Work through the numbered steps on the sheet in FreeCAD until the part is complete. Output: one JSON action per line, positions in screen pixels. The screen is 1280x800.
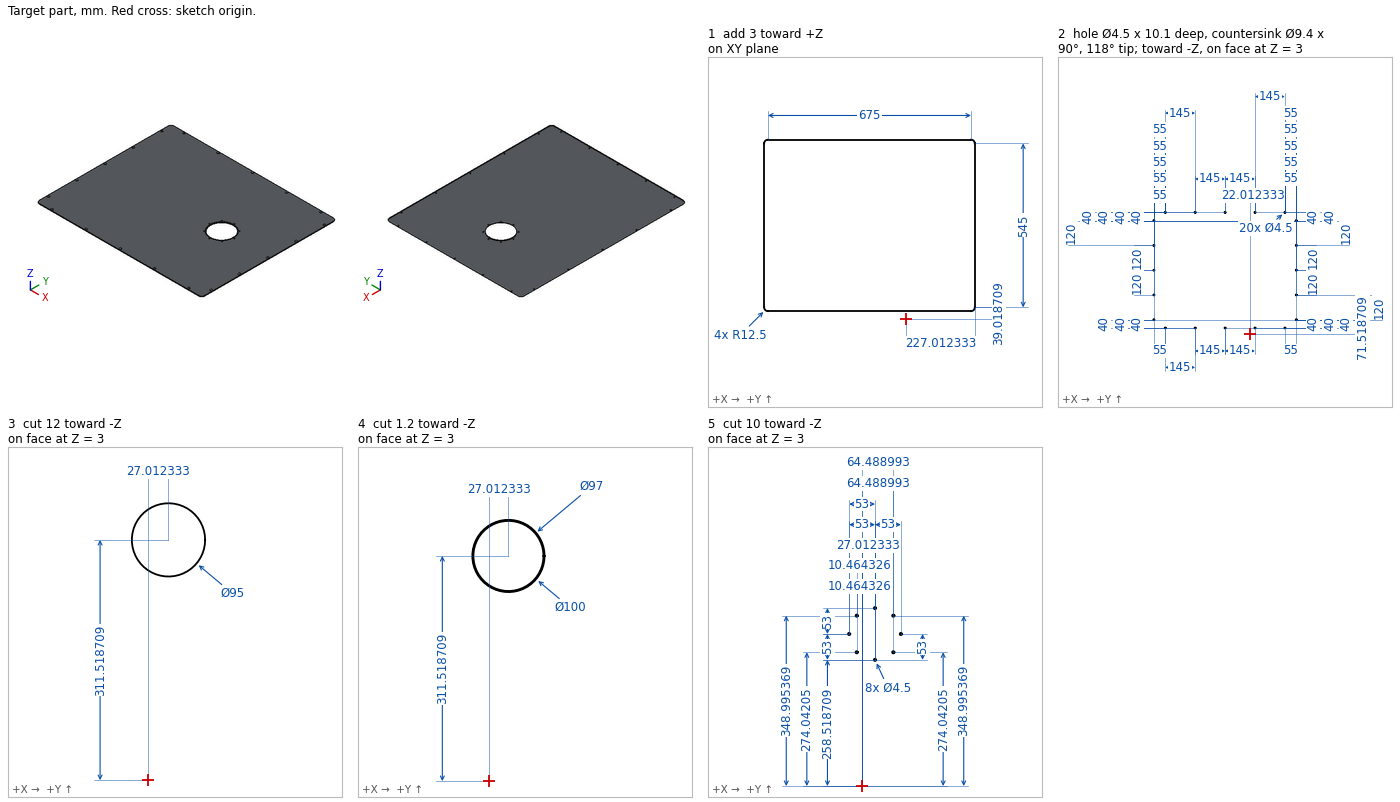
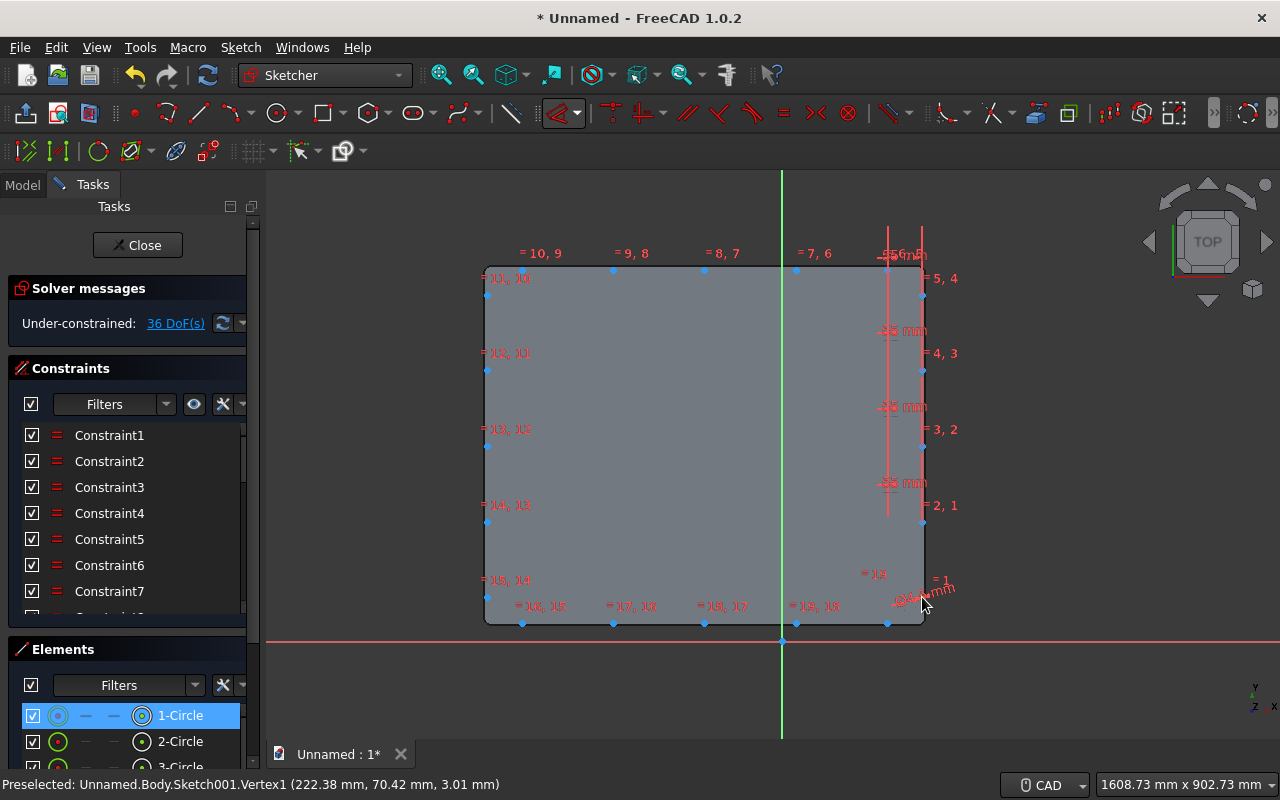
{"action": "left_click", "coordinate": [888, 270]}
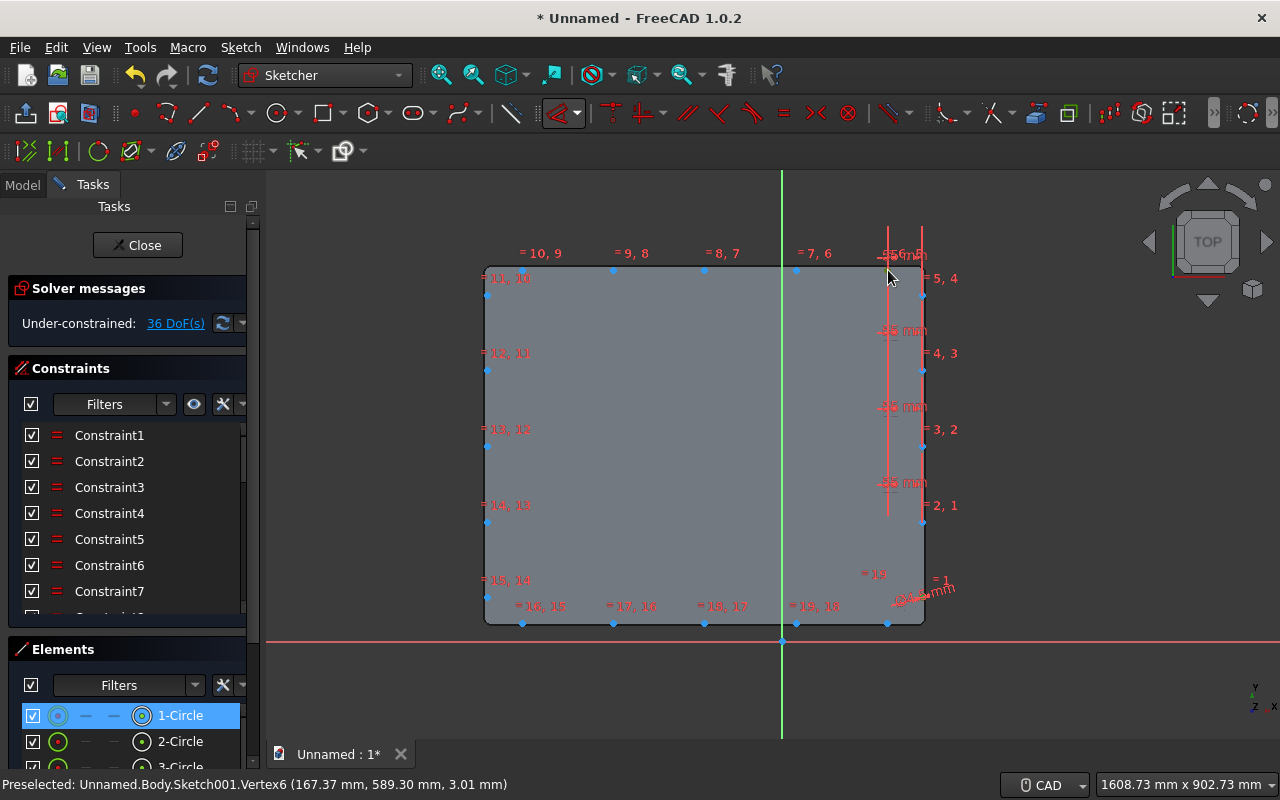
{"action": "key", "text": "l"}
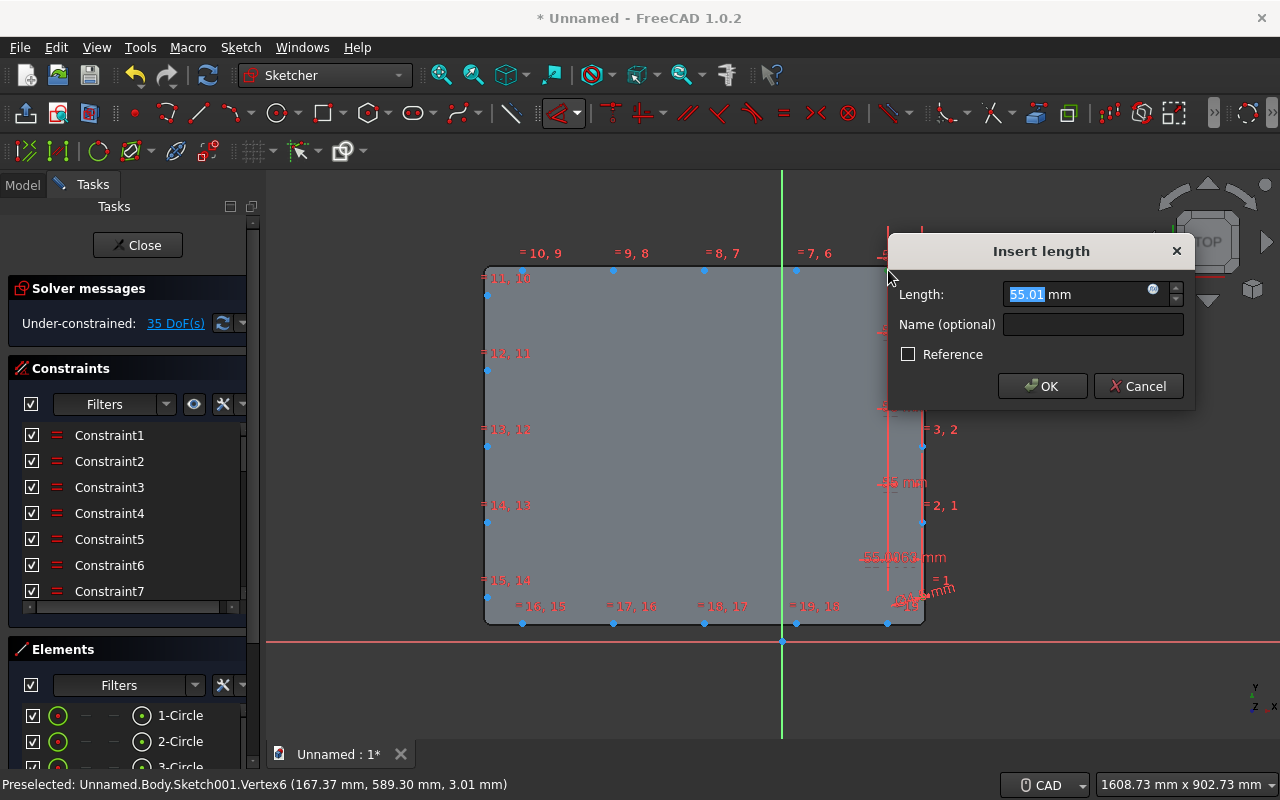
{"action": "type", "text": "55"}
{"action": "key", "text": "Return"}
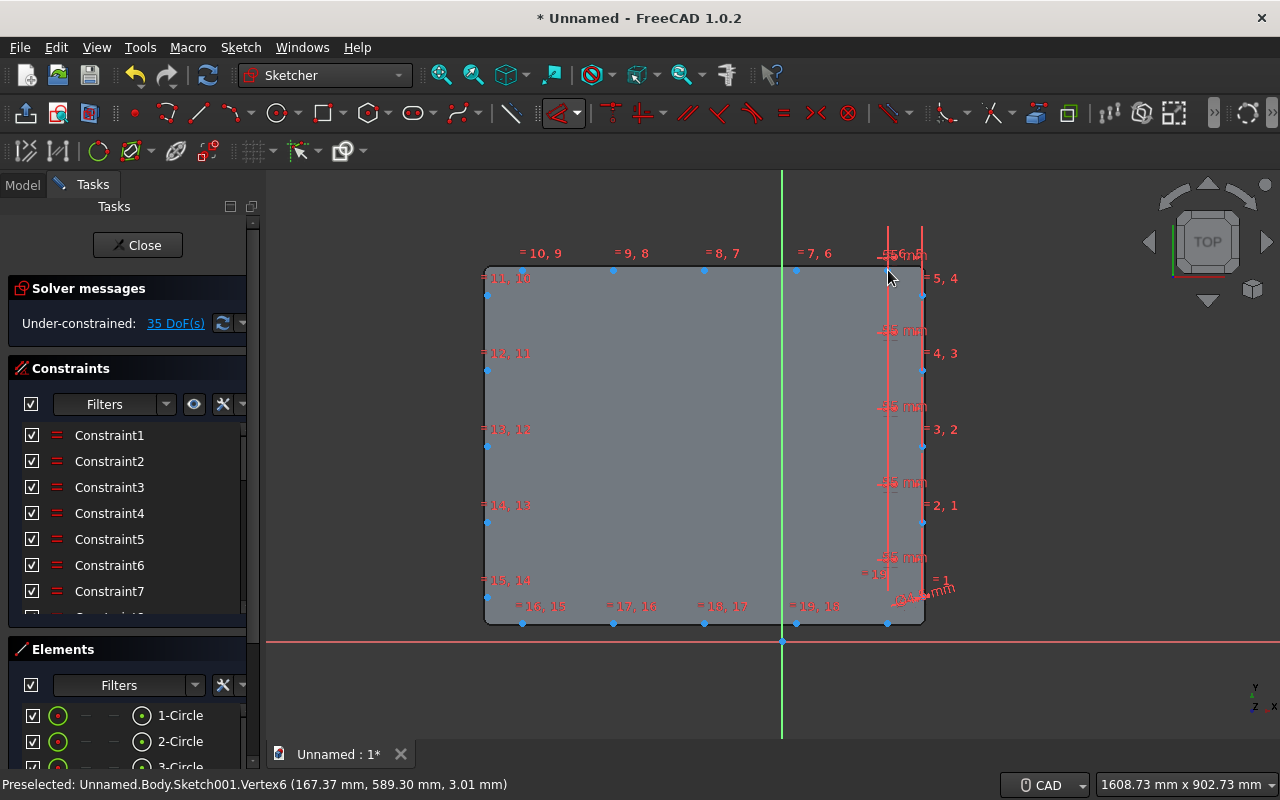
{"action": "scroll", "coordinate": [922, 295], "scroll_direction": "up", "scroll_amount": 3}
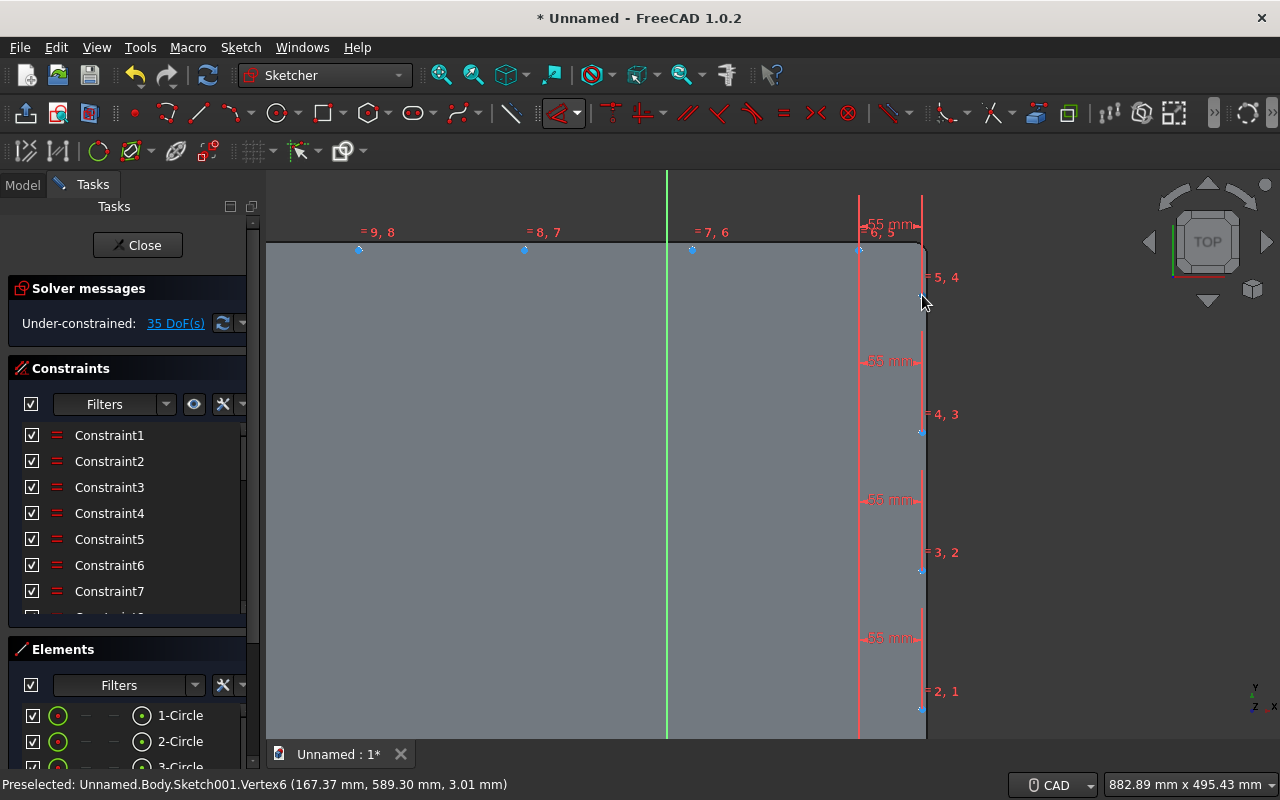
{"action": "left_click", "coordinate": [922, 296]}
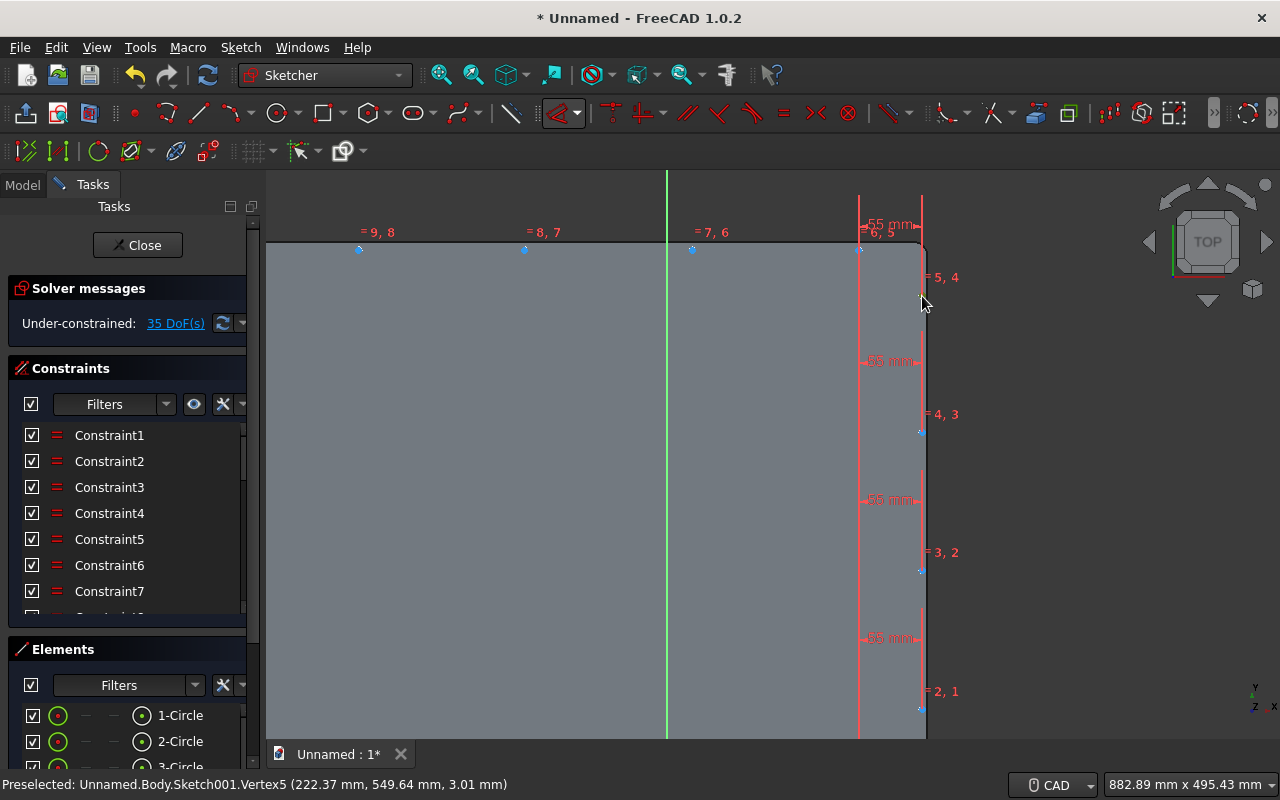
{"action": "left_click", "coordinate": [859, 250]}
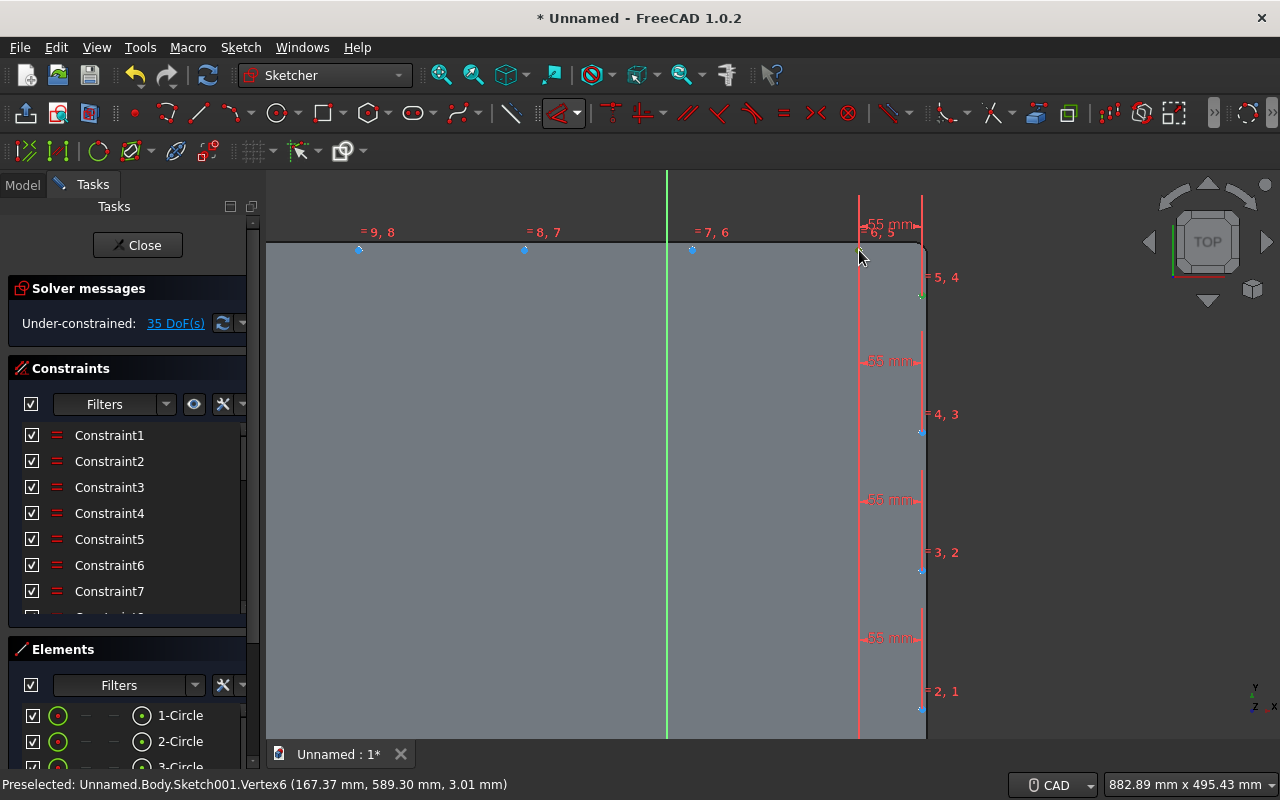
{"action": "left_click", "coordinate": [580, 114]}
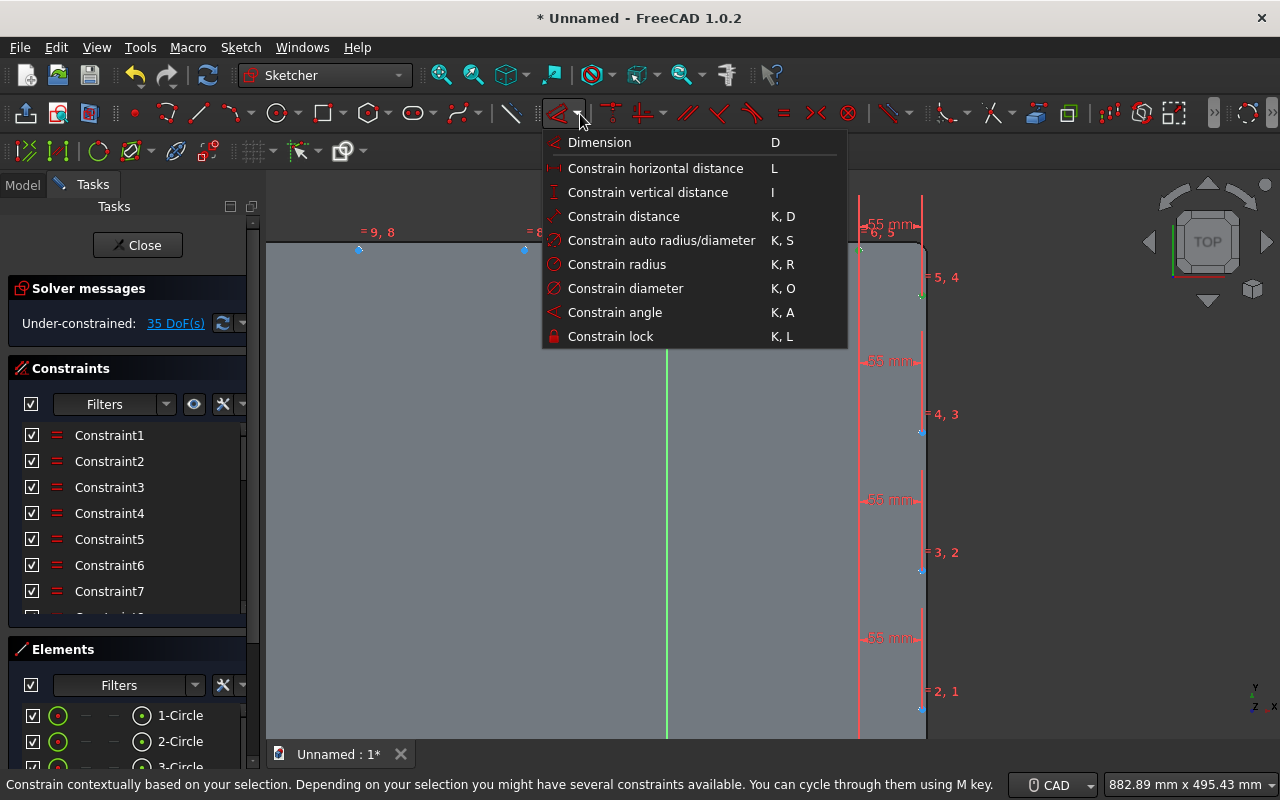
{"action": "left_click", "coordinate": [695, 192]}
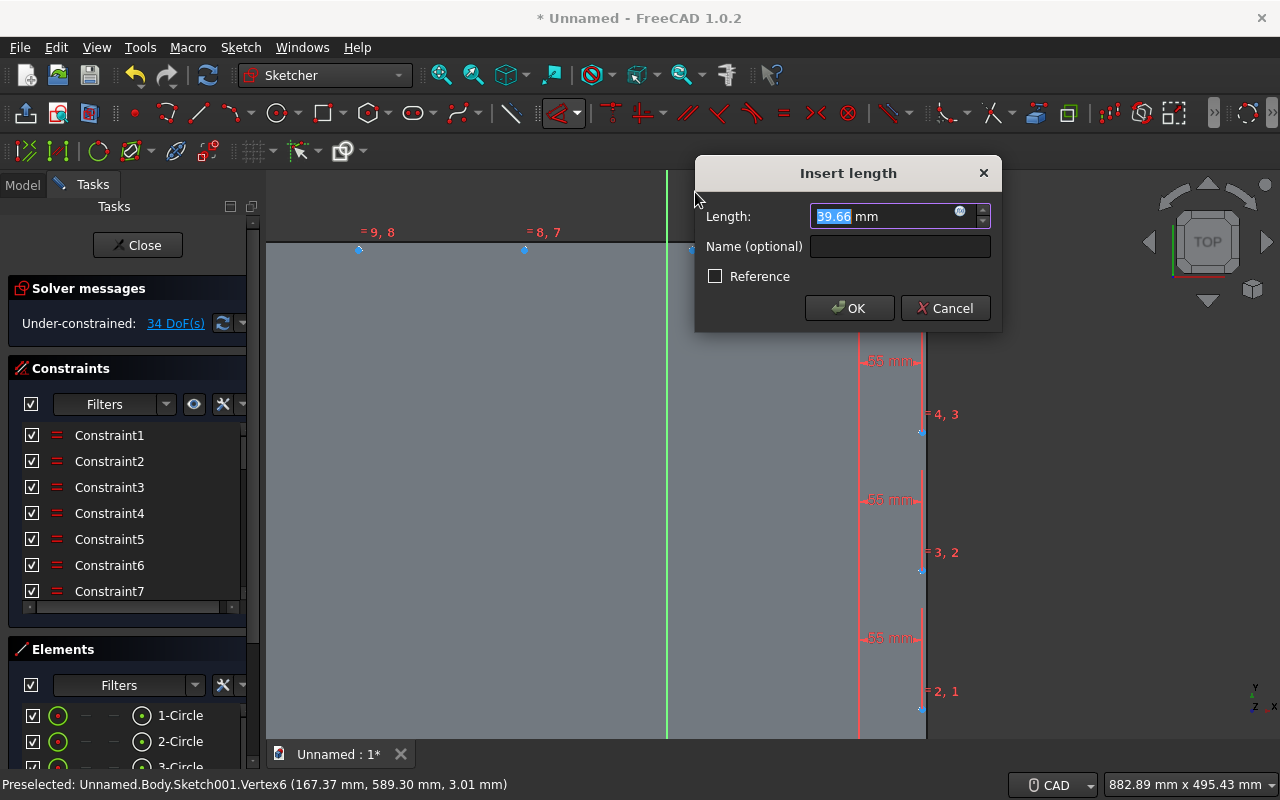
{"action": "type", "text": "40"}
{"action": "key", "text": "Return"}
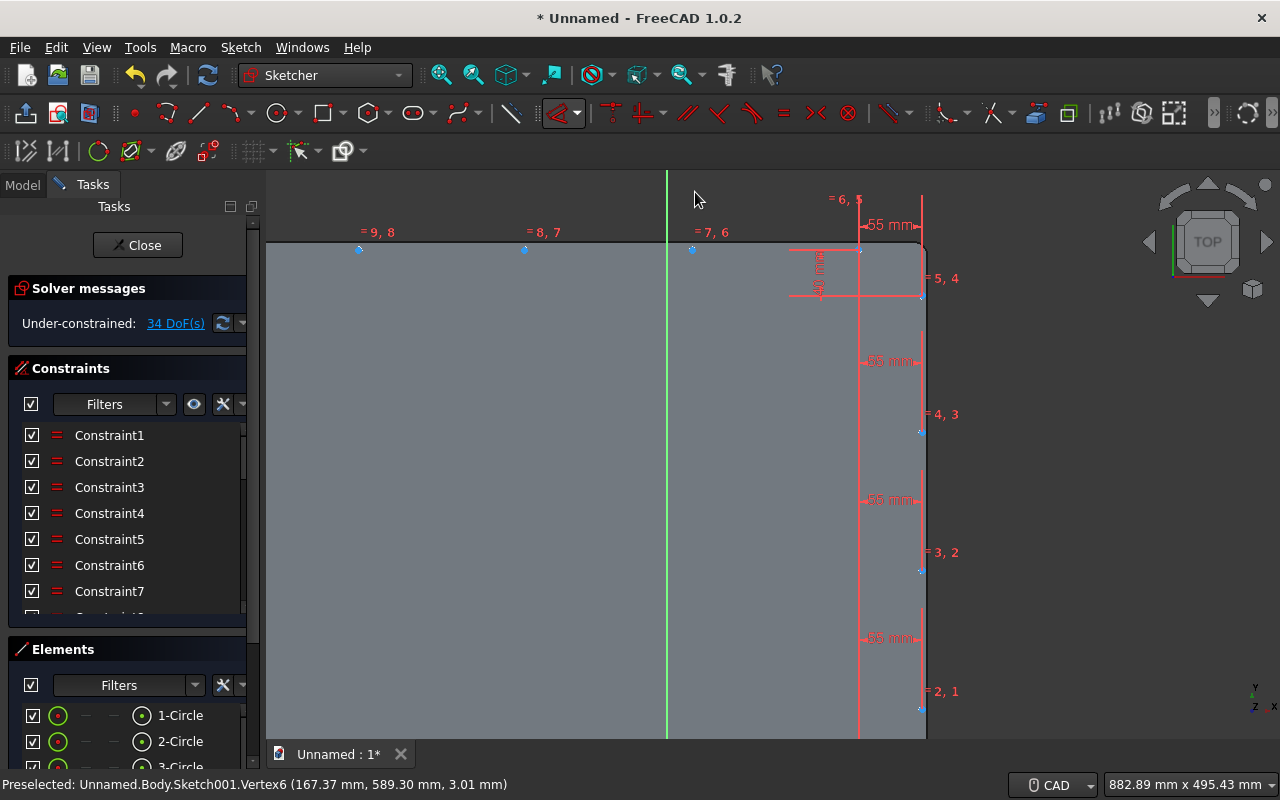
{"action": "left_click", "coordinate": [922, 296]}